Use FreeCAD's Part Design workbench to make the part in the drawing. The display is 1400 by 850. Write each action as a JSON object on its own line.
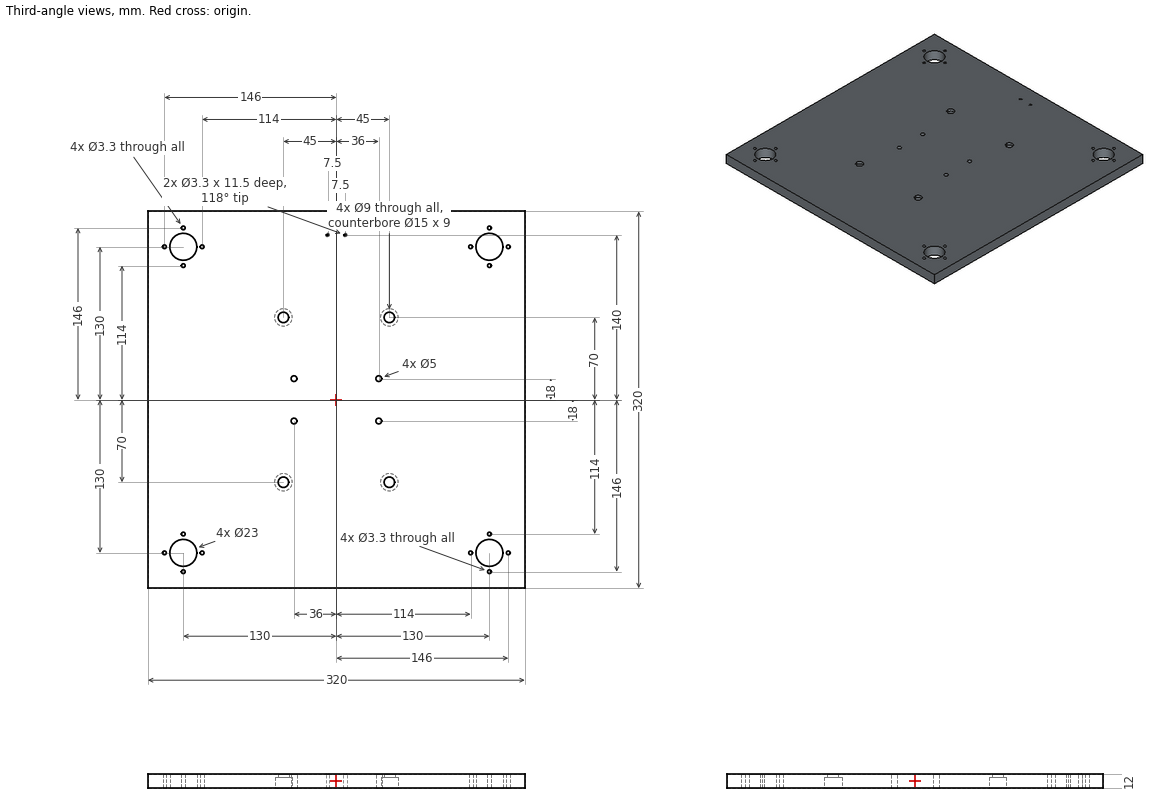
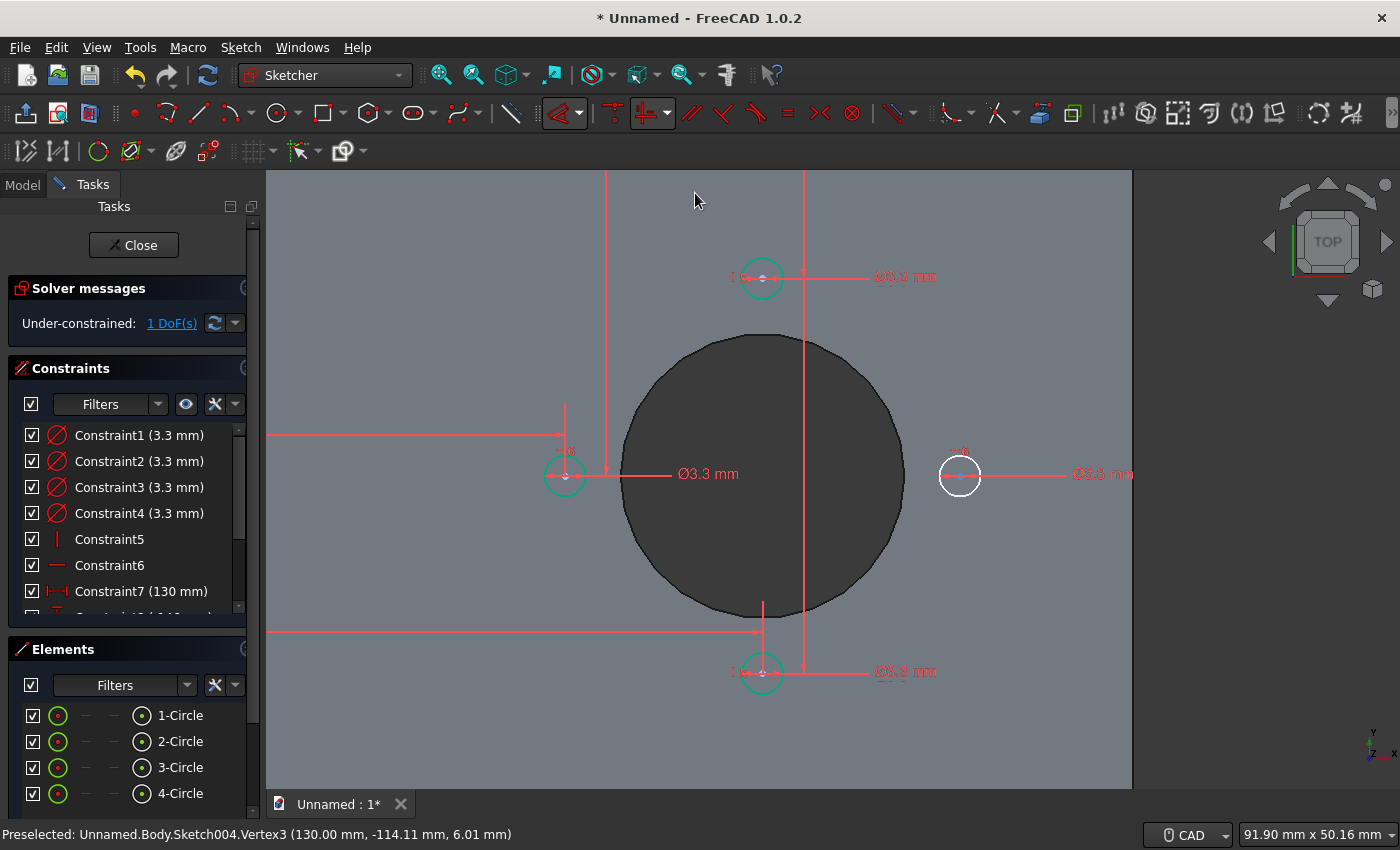
{"action": "left_click", "coordinate": [960, 476]}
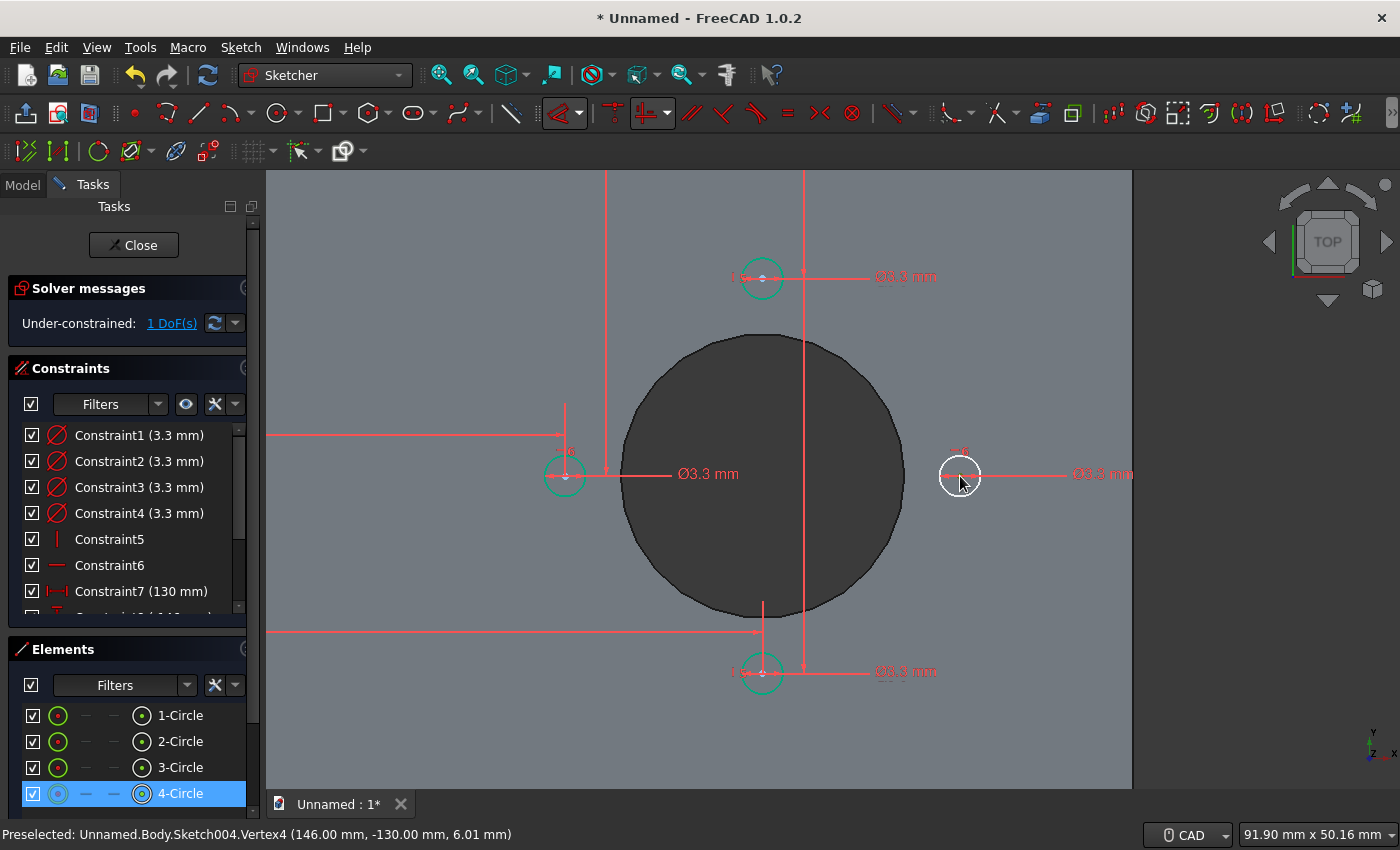
{"action": "left_click", "coordinate": [582, 114]}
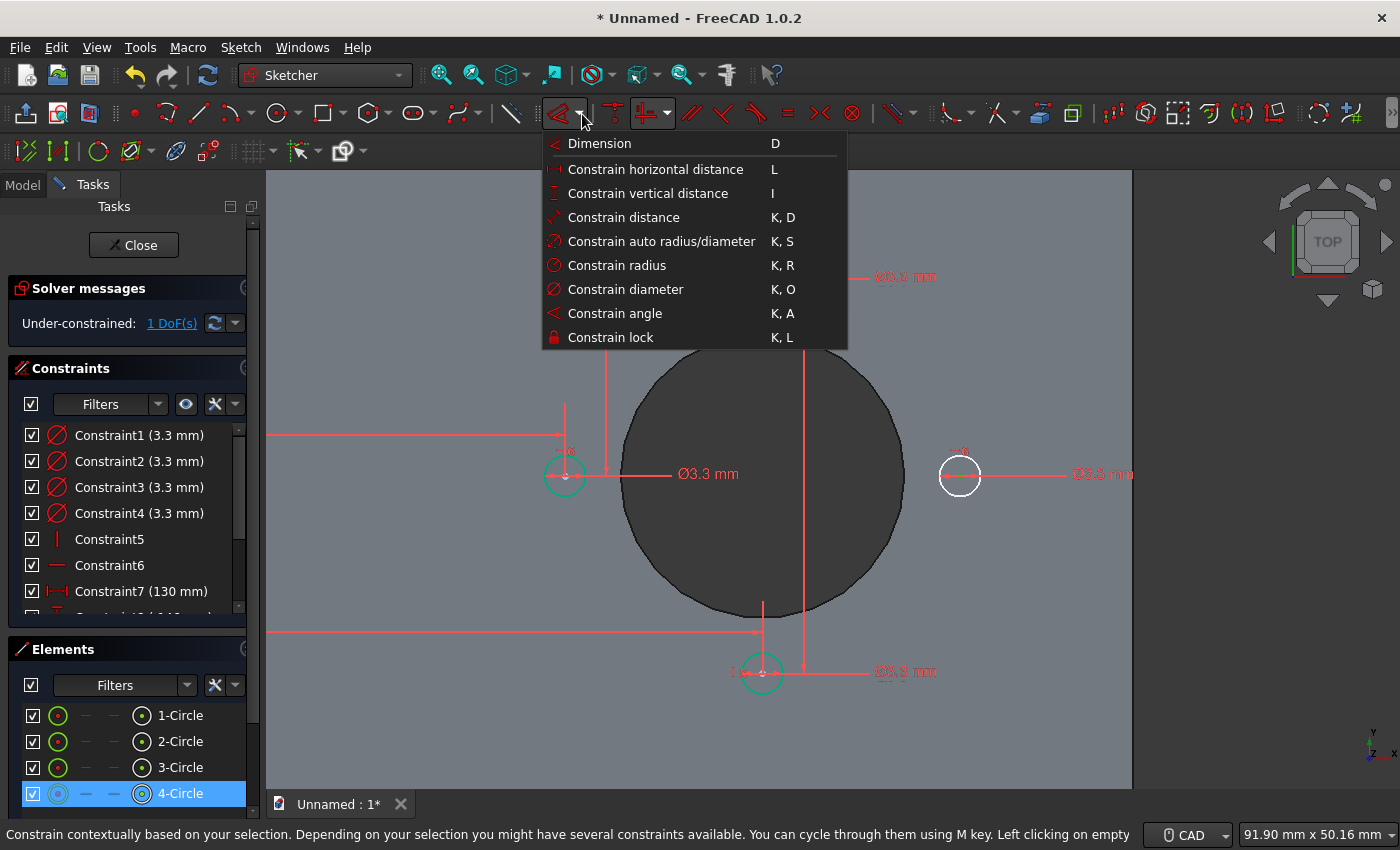
{"action": "left_click", "coordinate": [695, 169]}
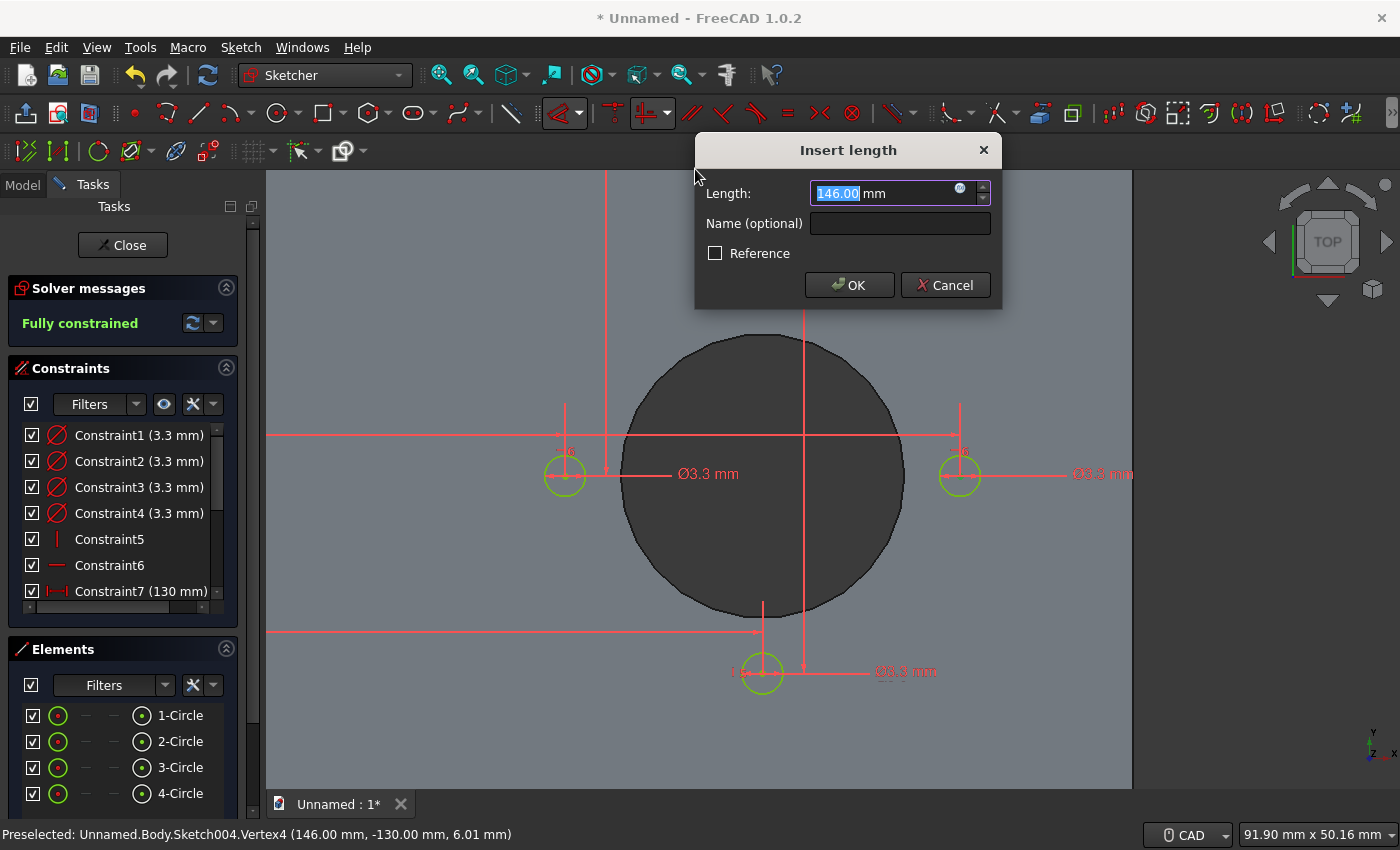
{"action": "type", "text": "146"}
{"action": "key", "text": "Return"}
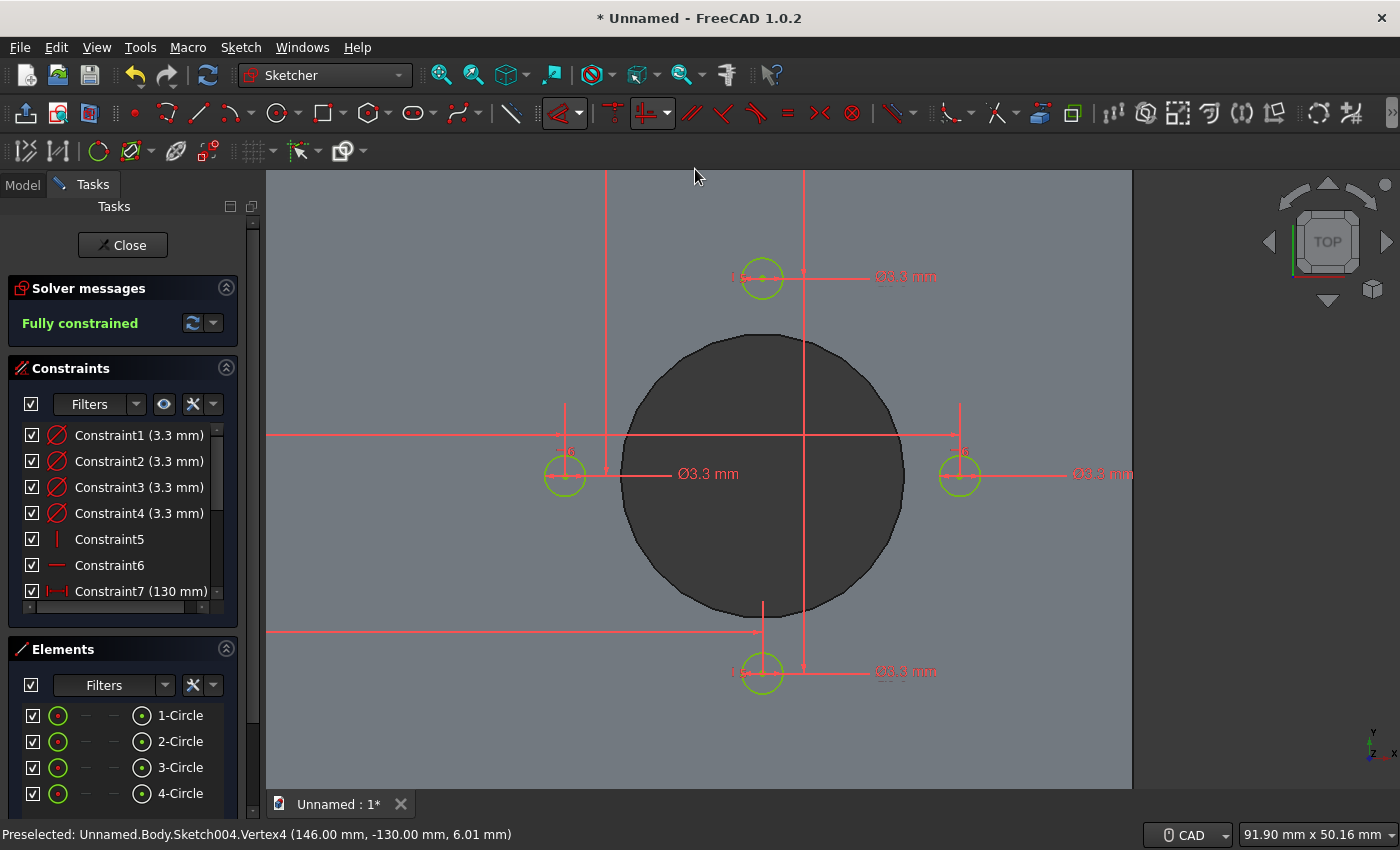
{"action": "left_click", "coordinate": [123, 245]}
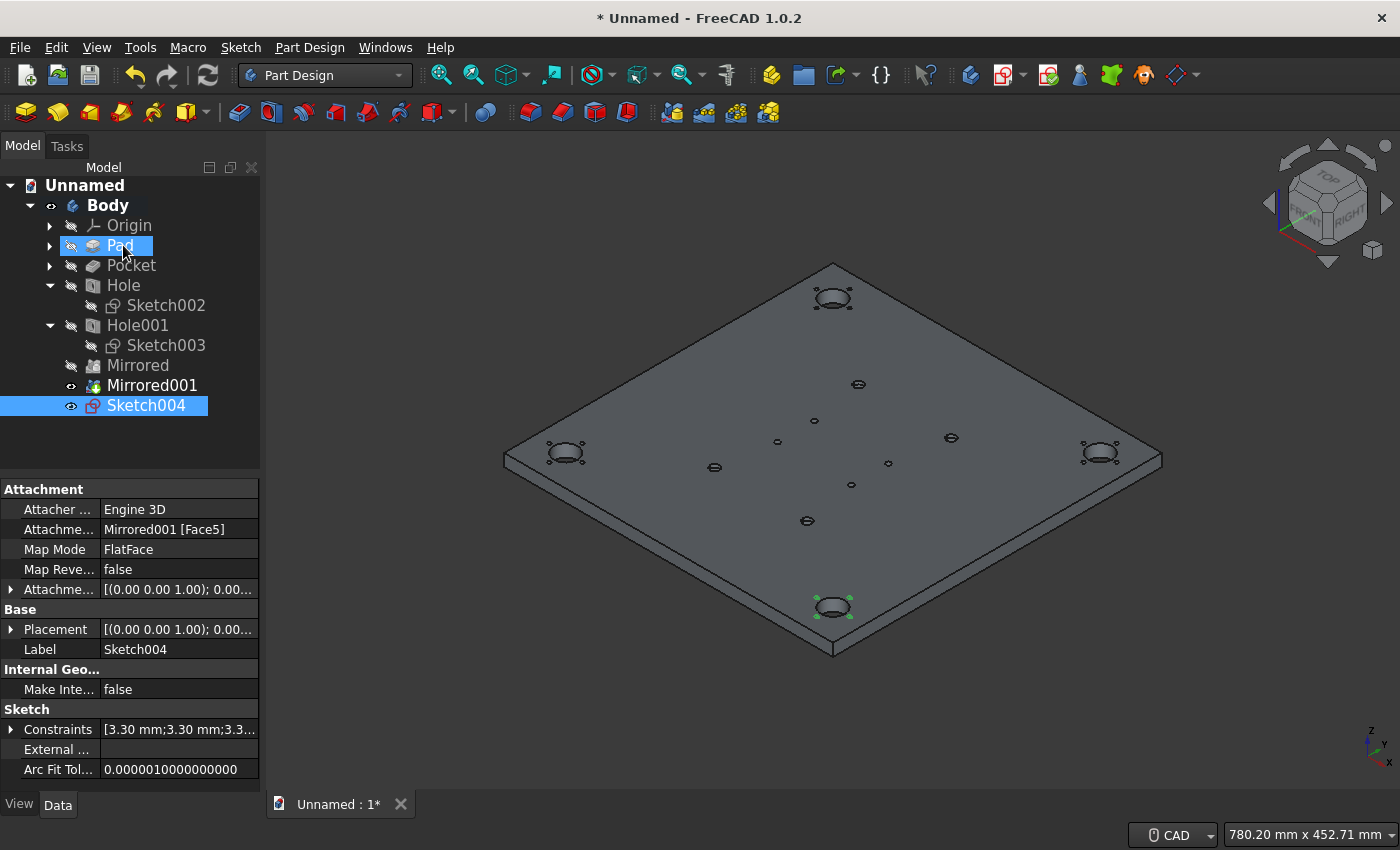
{"action": "left_click", "coordinate": [272, 112]}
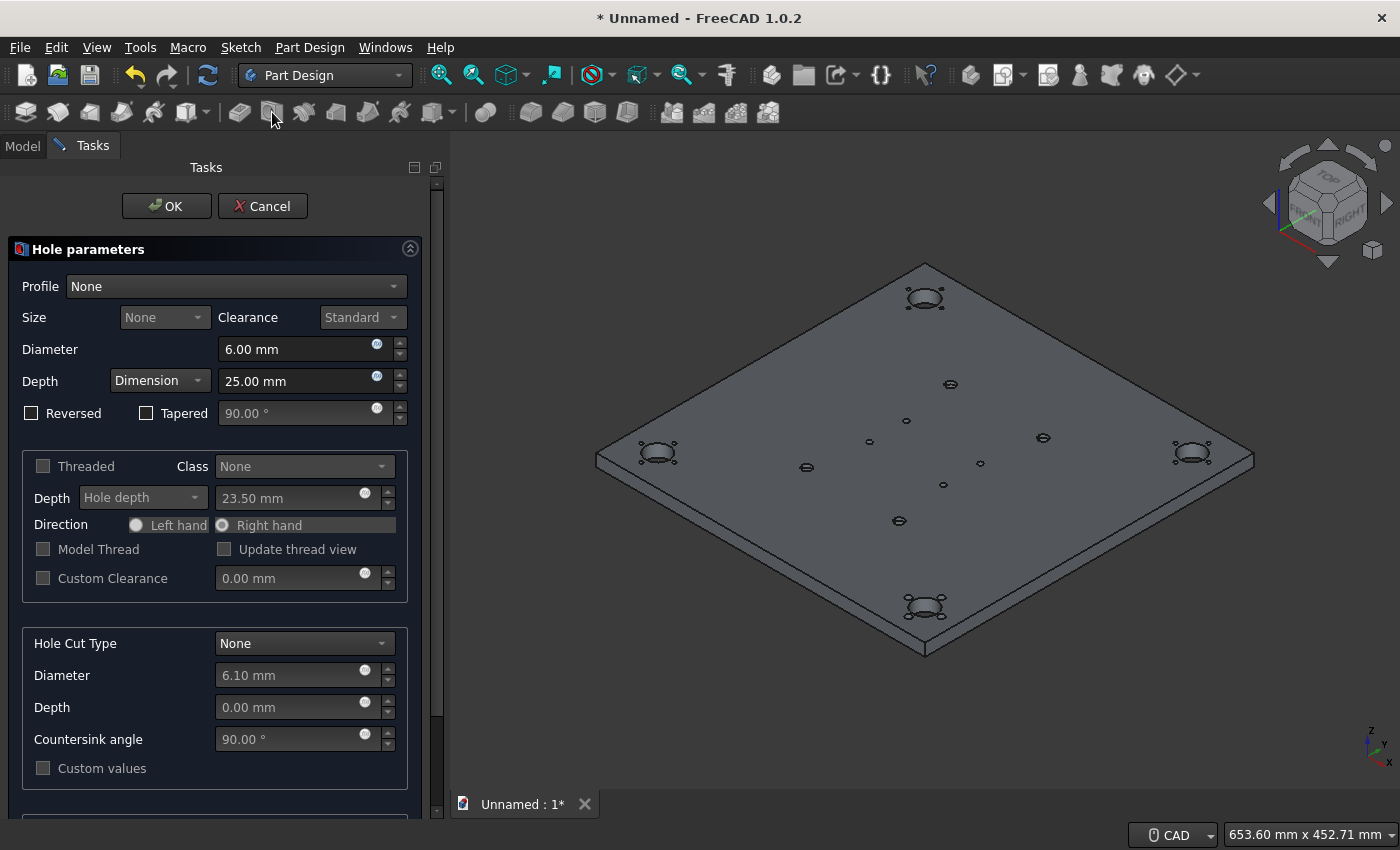
{"action": "triple_click", "coordinate": [305, 349]}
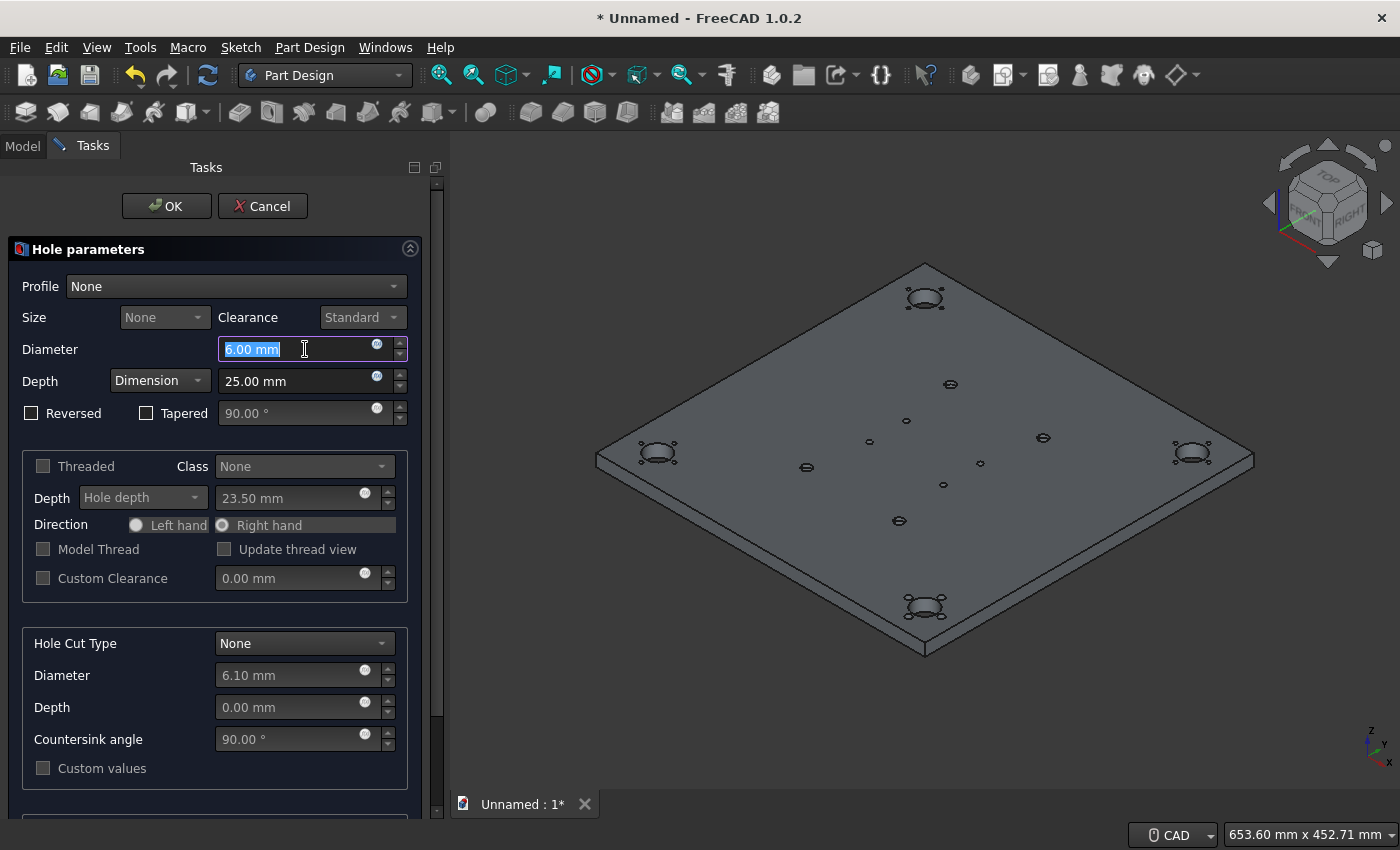
{"action": "type", "text": "3.3"}
{"action": "key", "text": "Tab"}